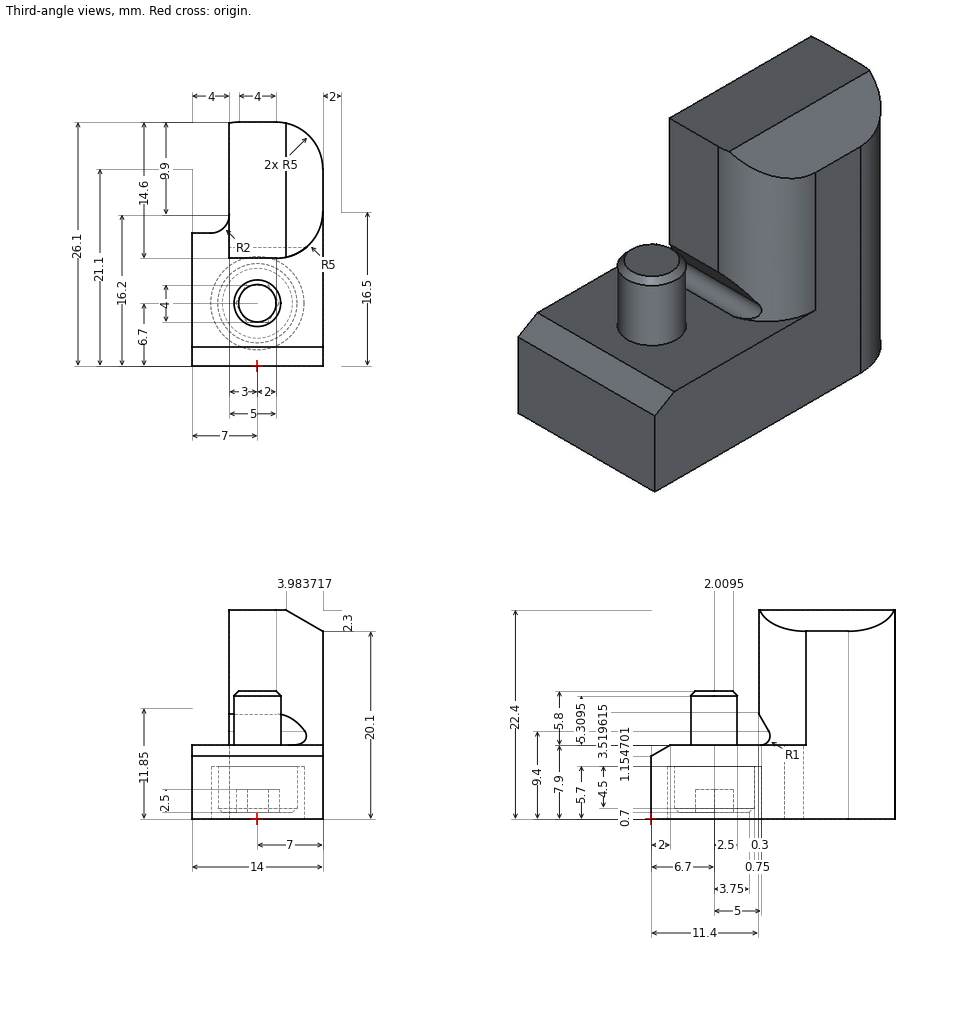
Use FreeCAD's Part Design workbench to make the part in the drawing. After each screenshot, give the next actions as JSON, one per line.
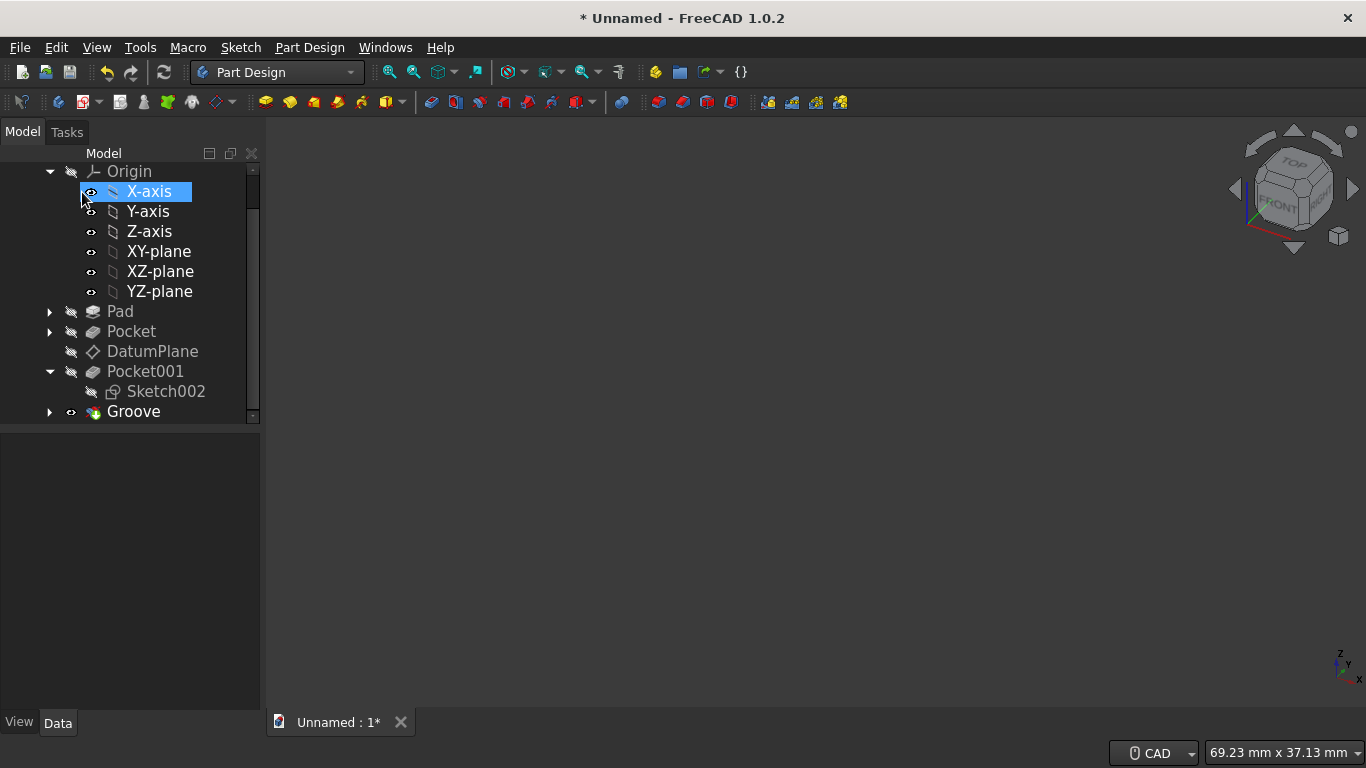
{"action": "left_click", "coordinate": [390, 72]}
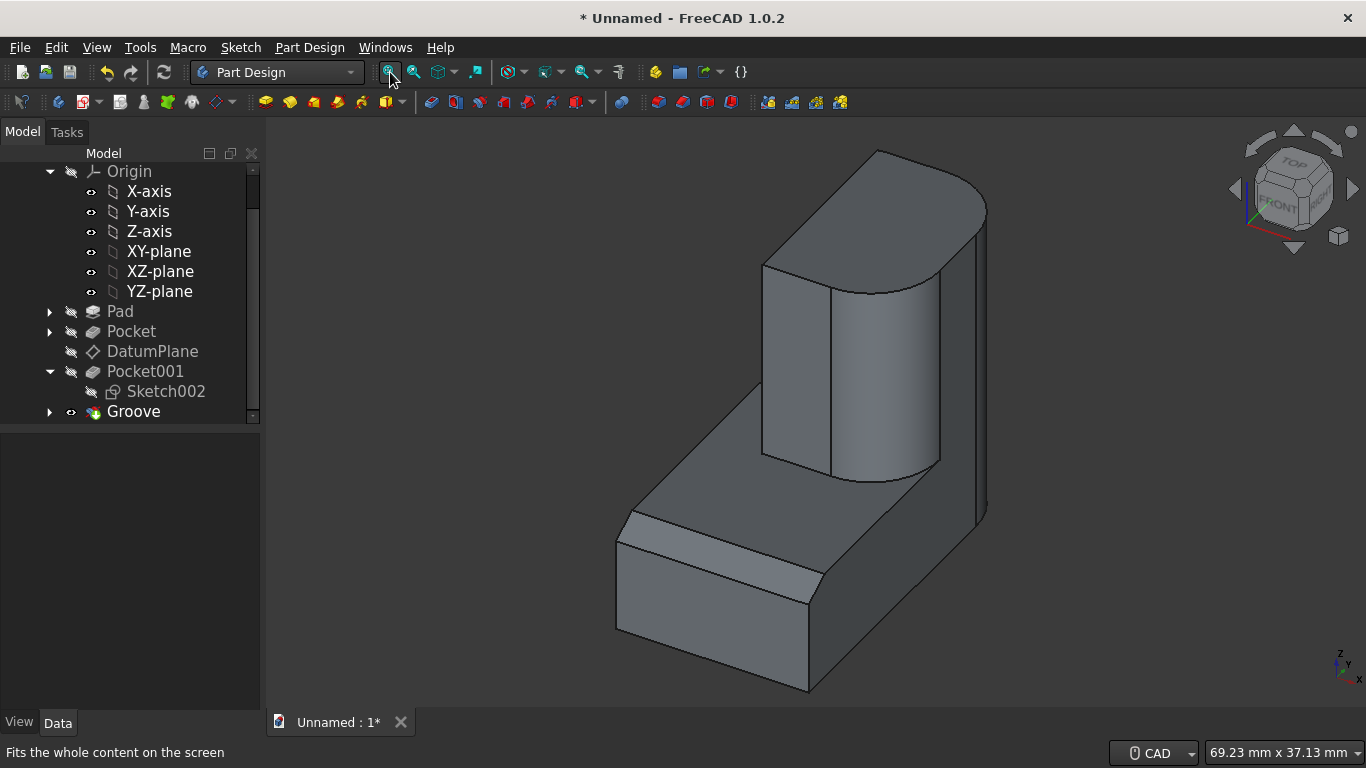
{"action": "key", "text": "5"}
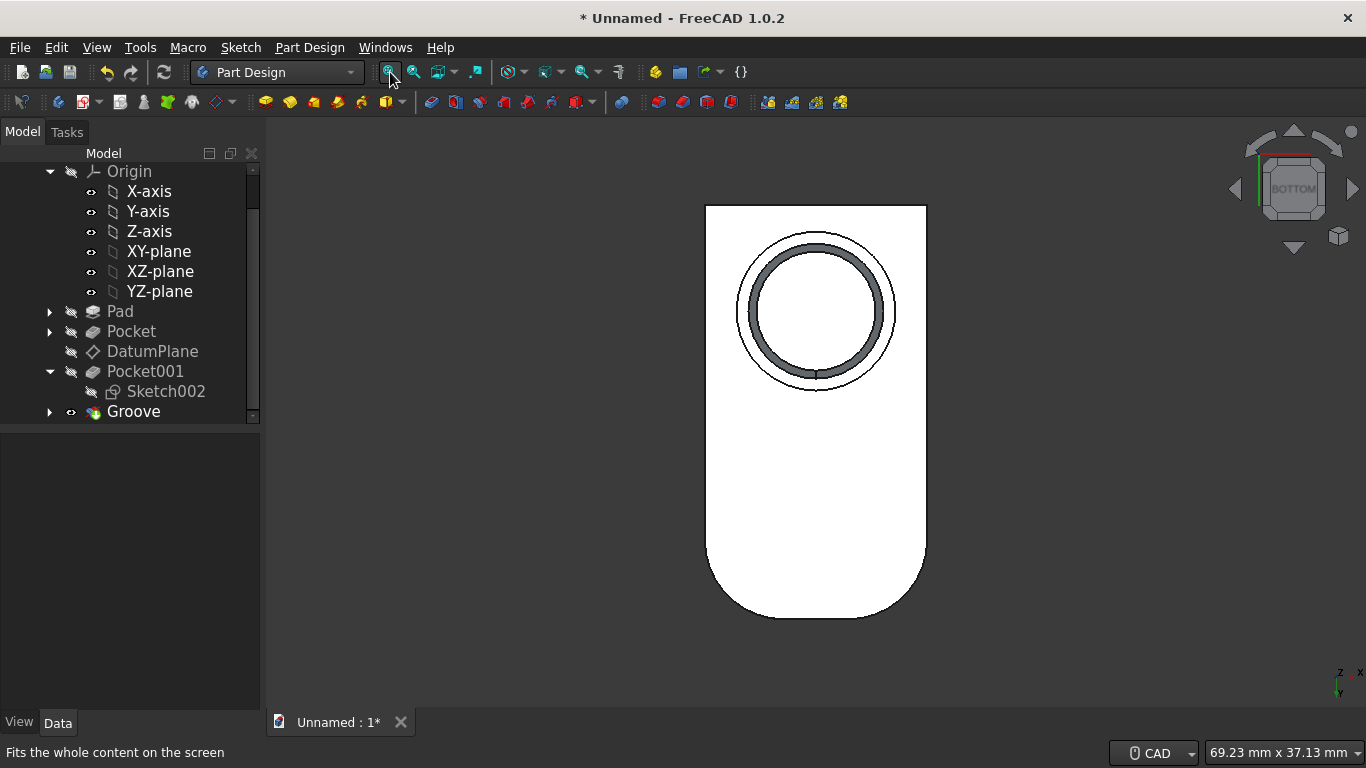
{"action": "left_click", "coordinate": [816, 310]}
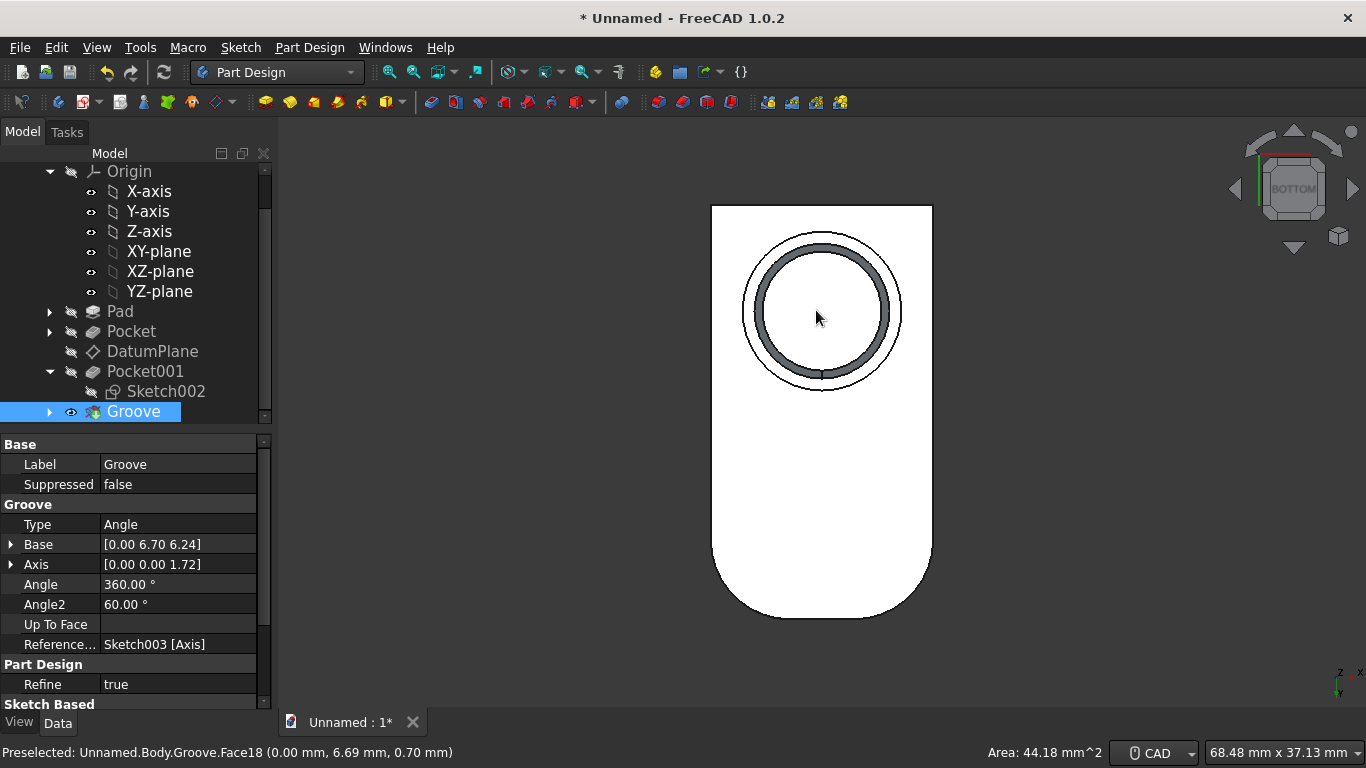
{"action": "left_click", "coordinate": [84, 102]}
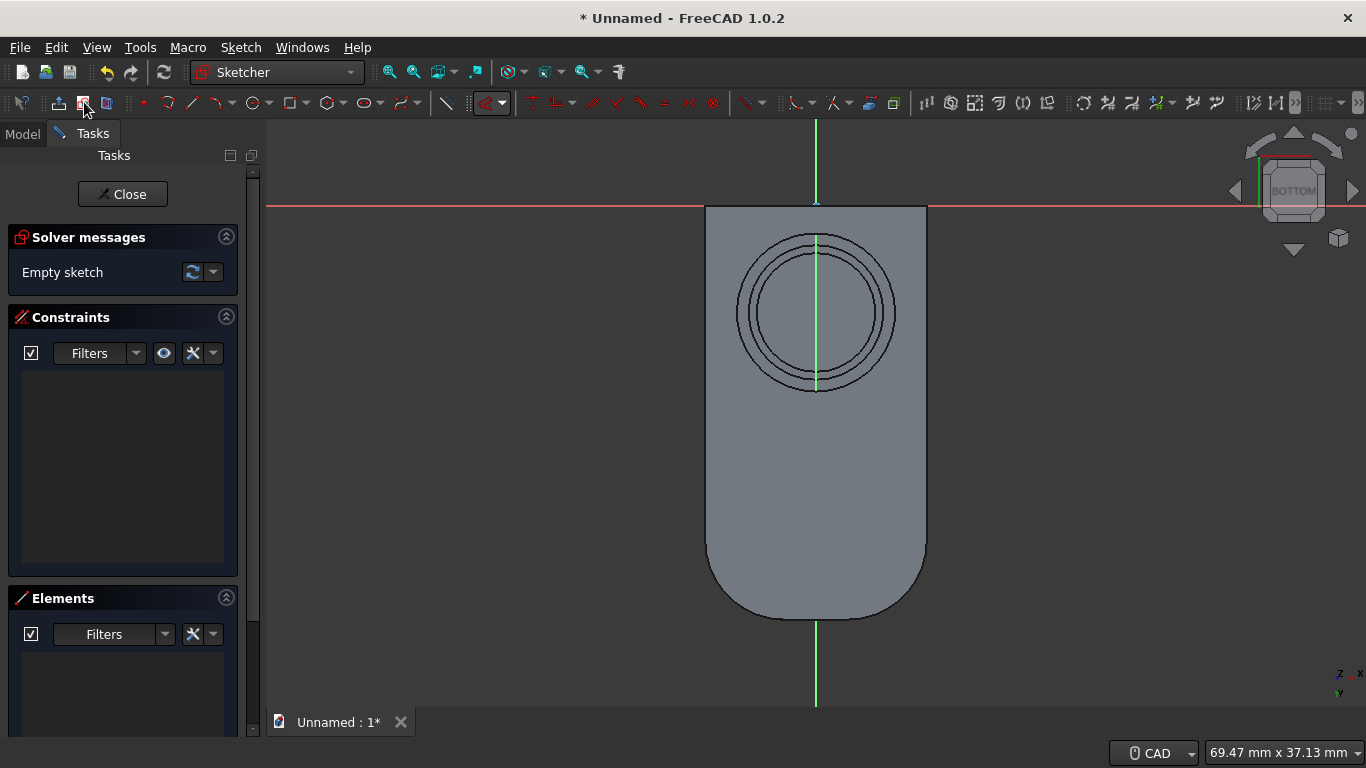
{"action": "left_click", "coordinate": [108, 104]}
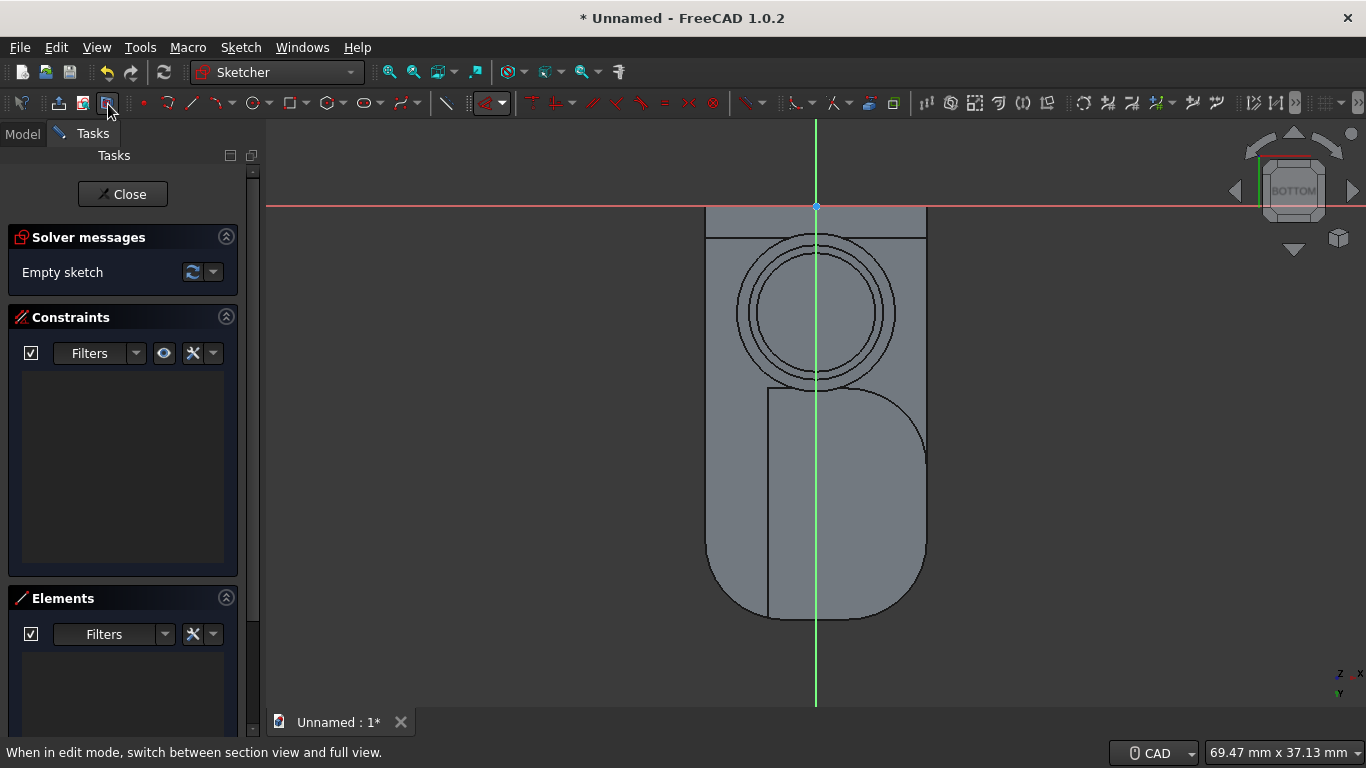
{"action": "scroll", "coordinate": [856, 195], "scroll_direction": "up", "scroll_amount": 5}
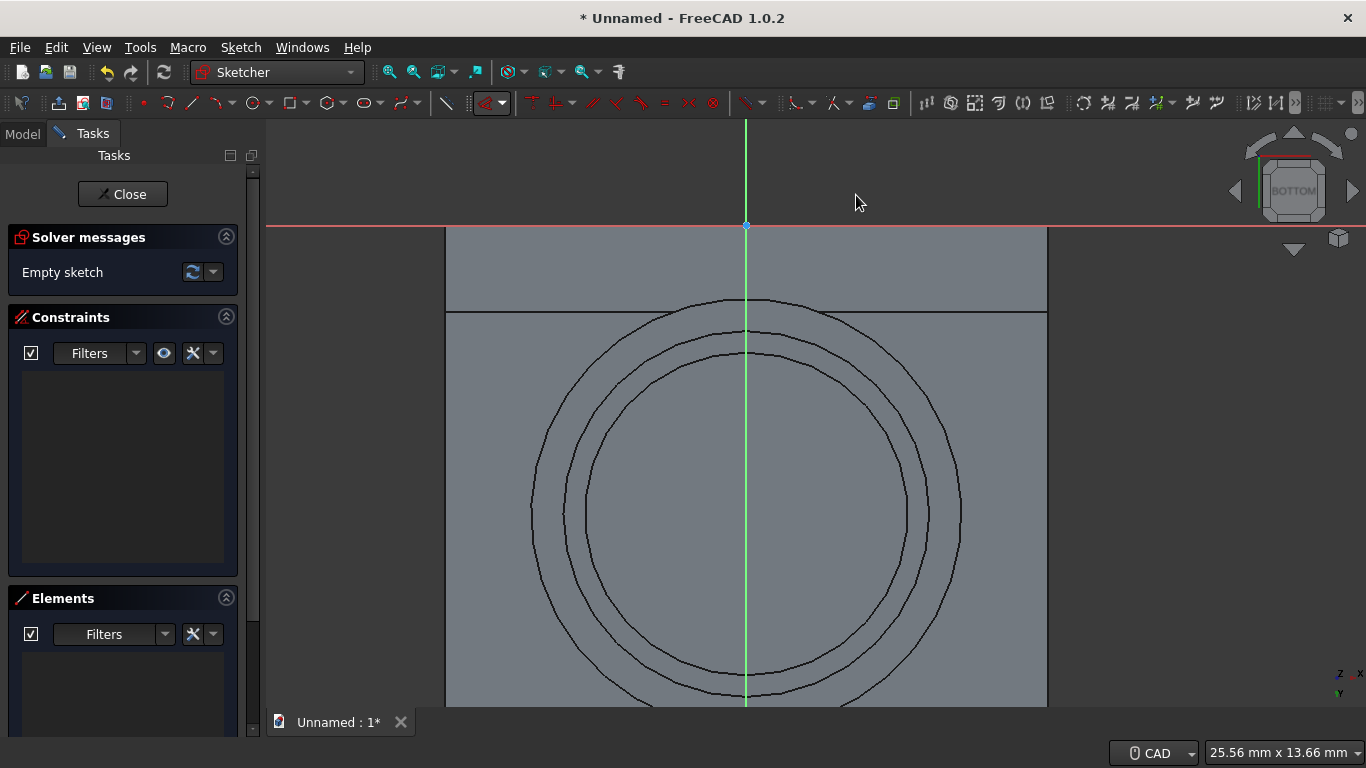
{"action": "left_click", "coordinate": [328, 104]}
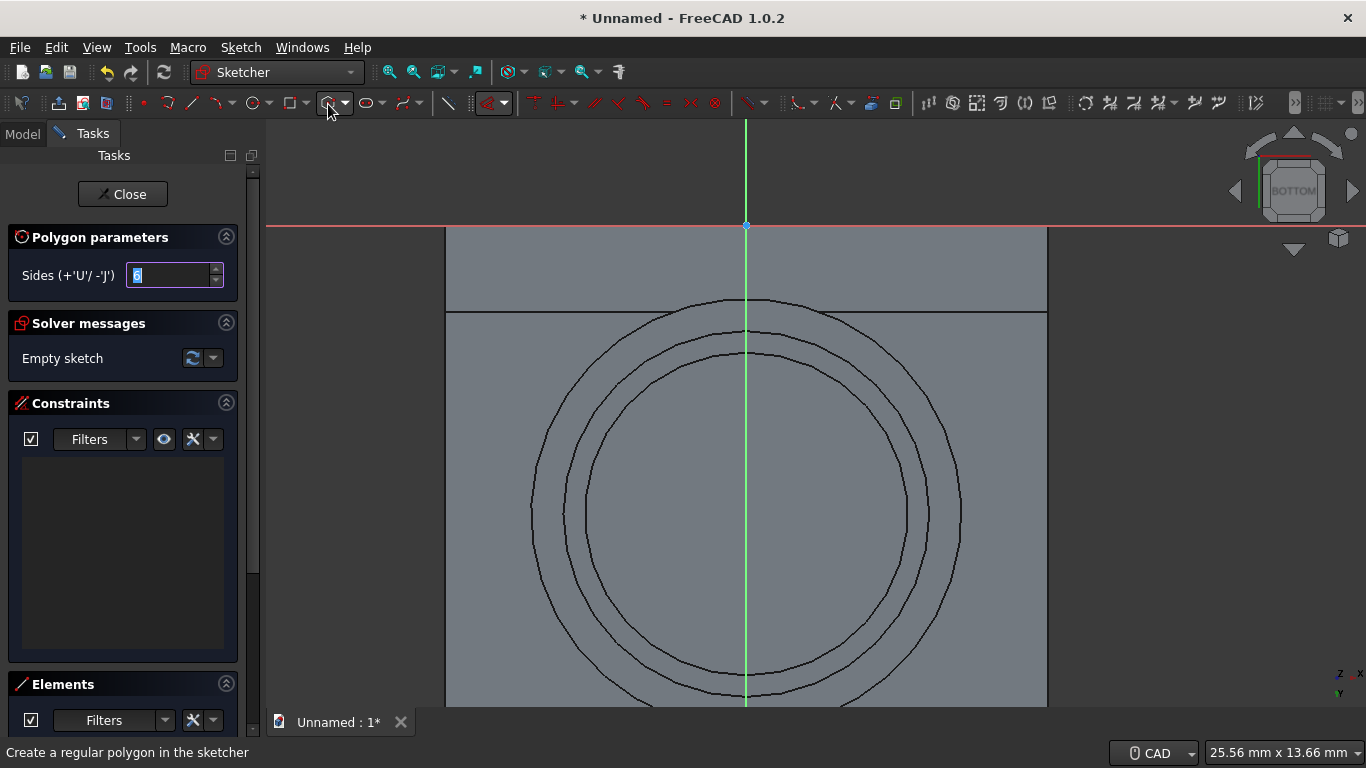
{"action": "left_click", "coordinate": [746, 514]}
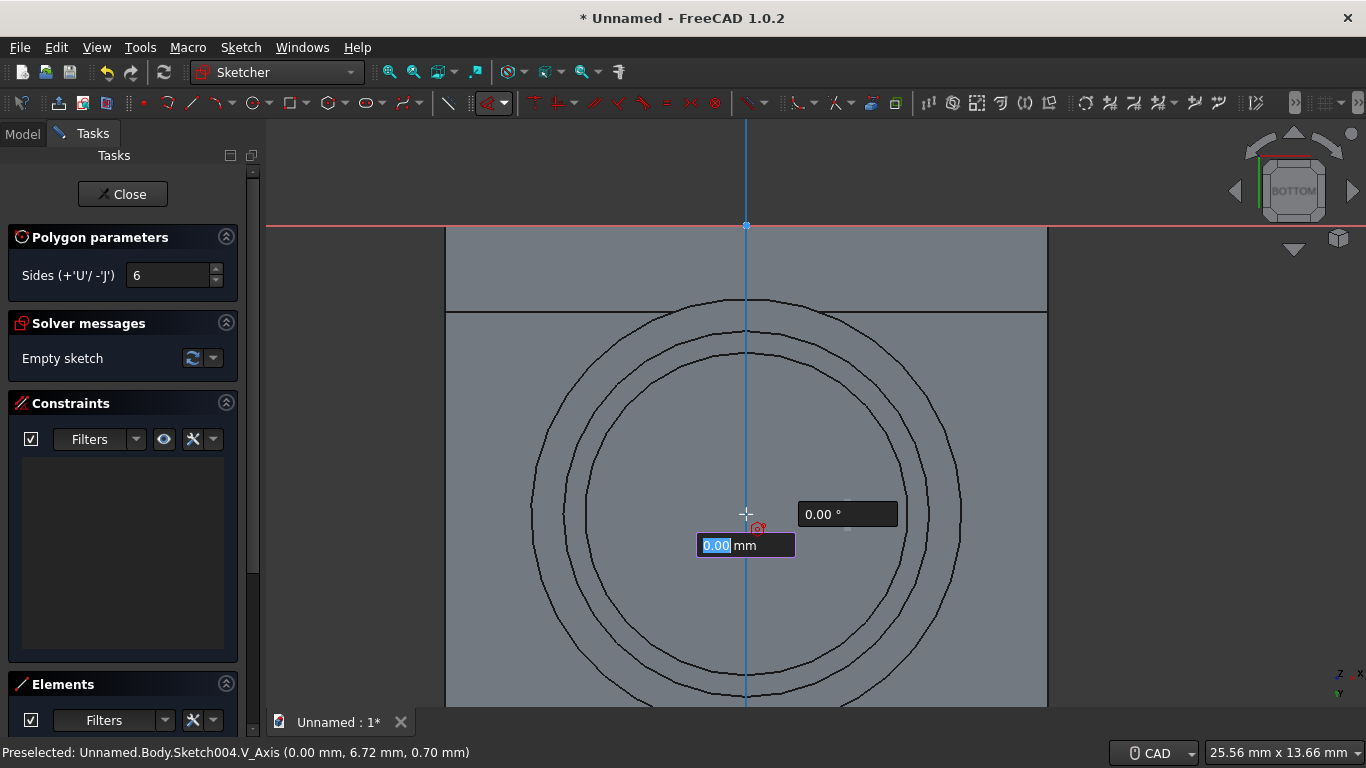
{"action": "left_click", "coordinate": [647, 514]}
{"action": "right_click", "coordinate": [647, 514]}